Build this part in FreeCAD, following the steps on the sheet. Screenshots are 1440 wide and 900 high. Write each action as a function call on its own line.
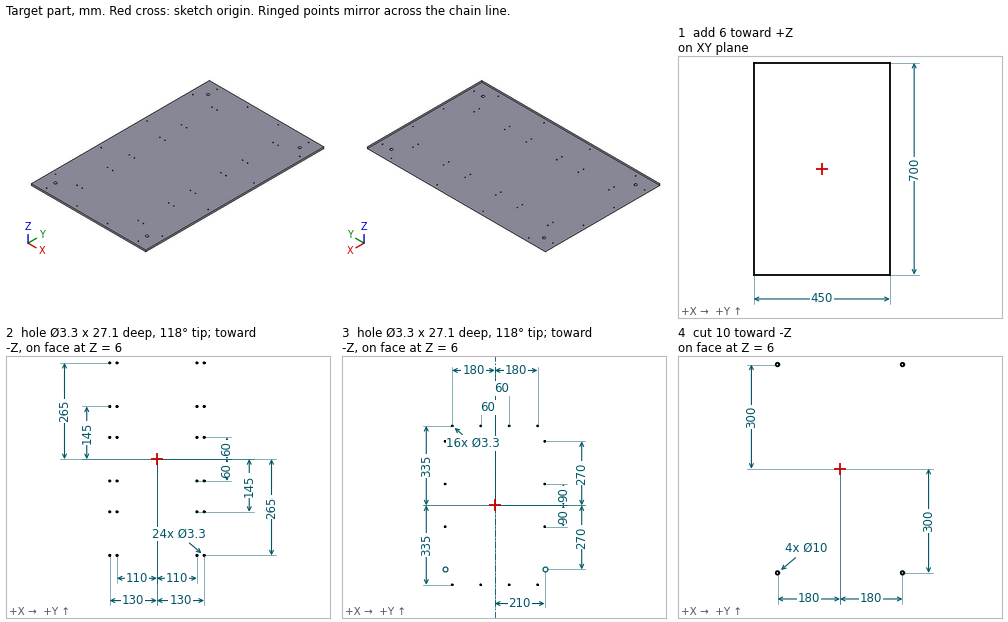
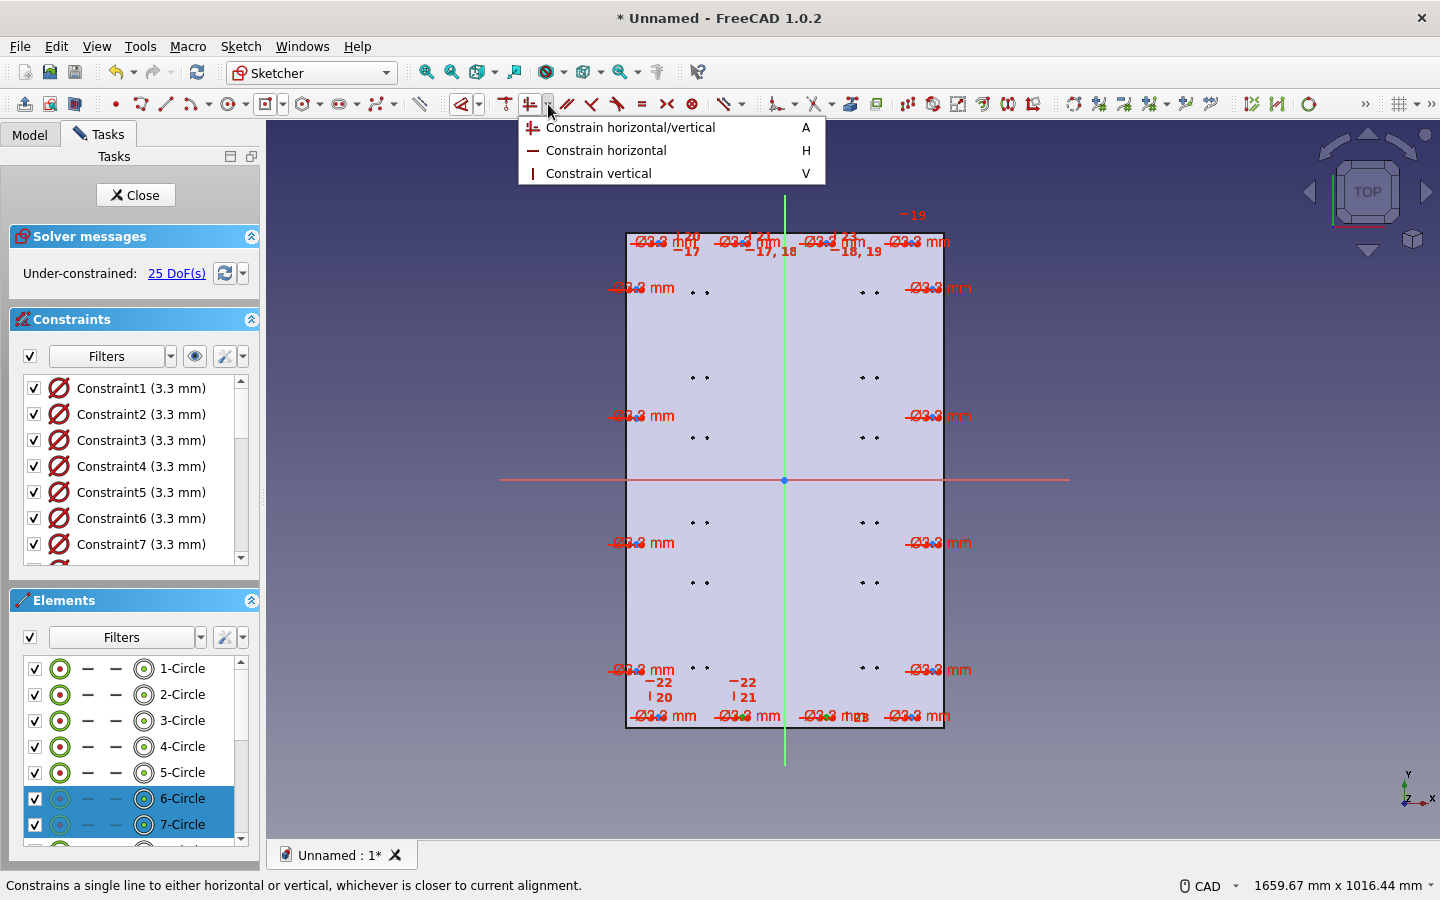
click(672, 150)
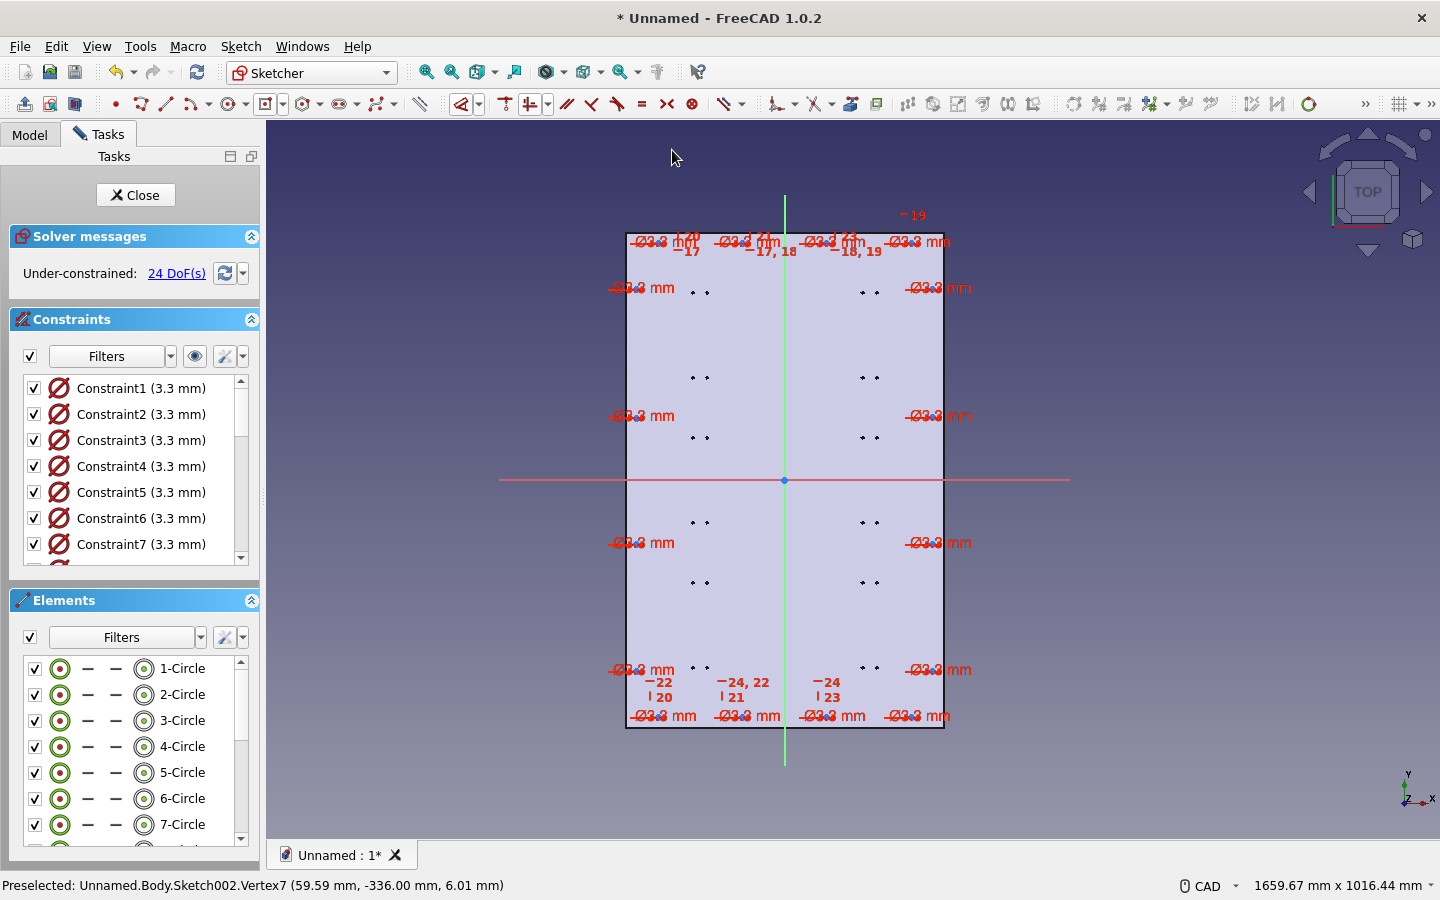
click(912, 244)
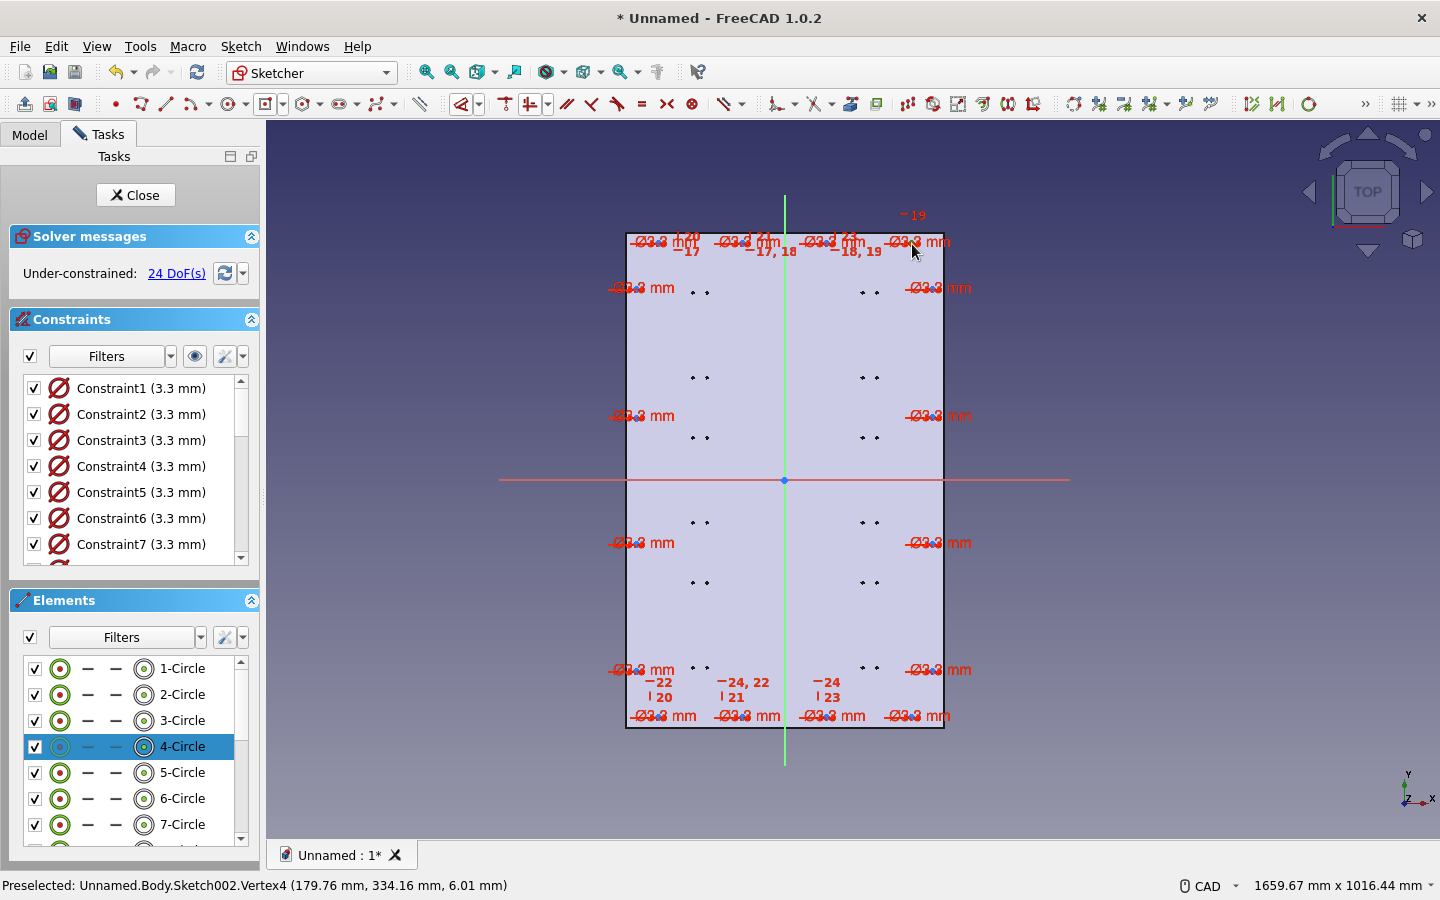
click(912, 718)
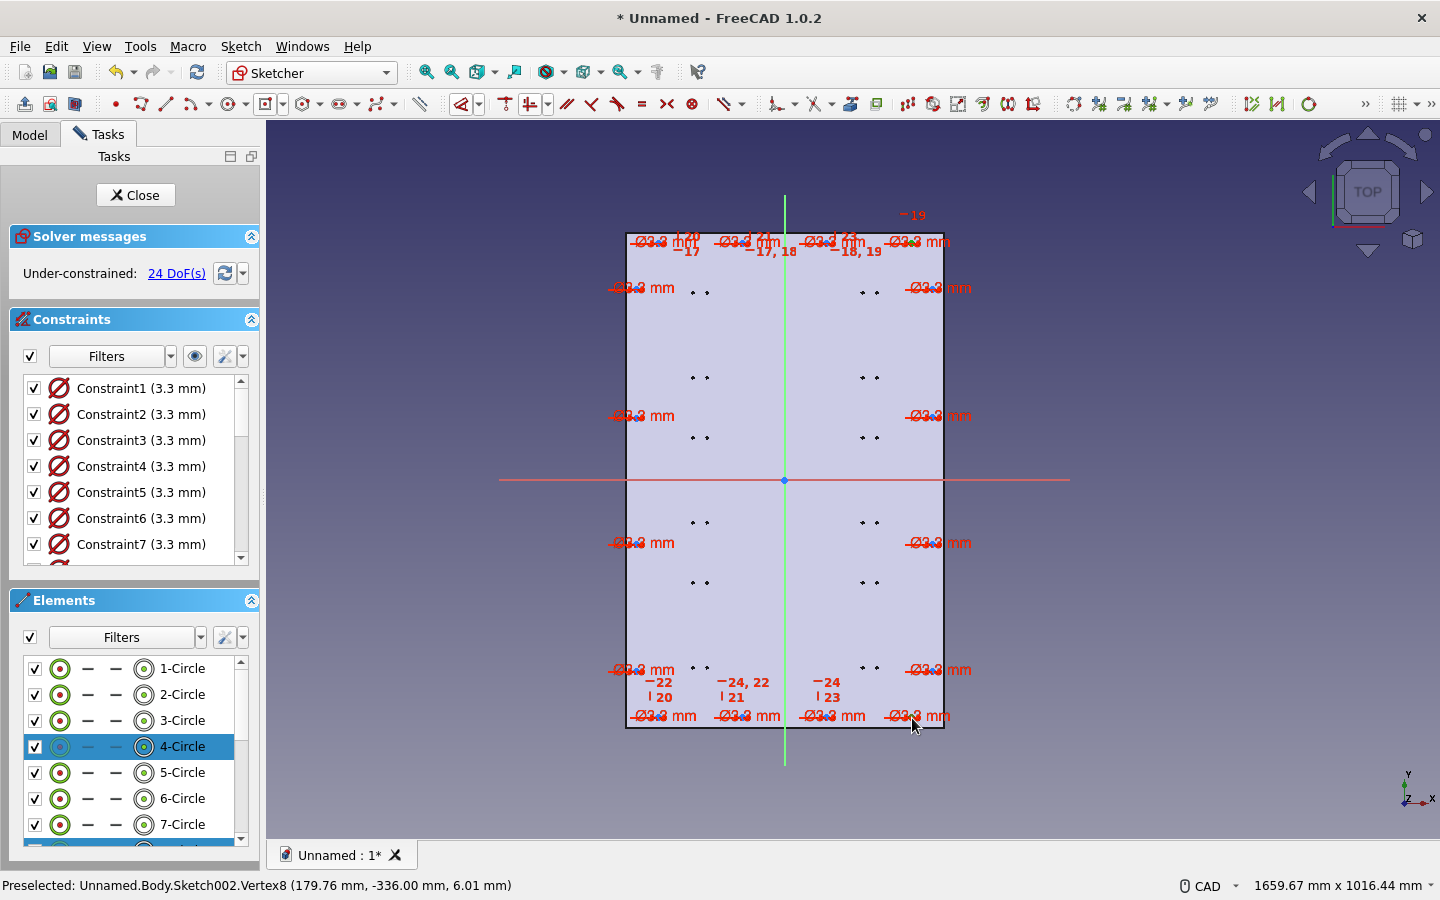
click(548, 104)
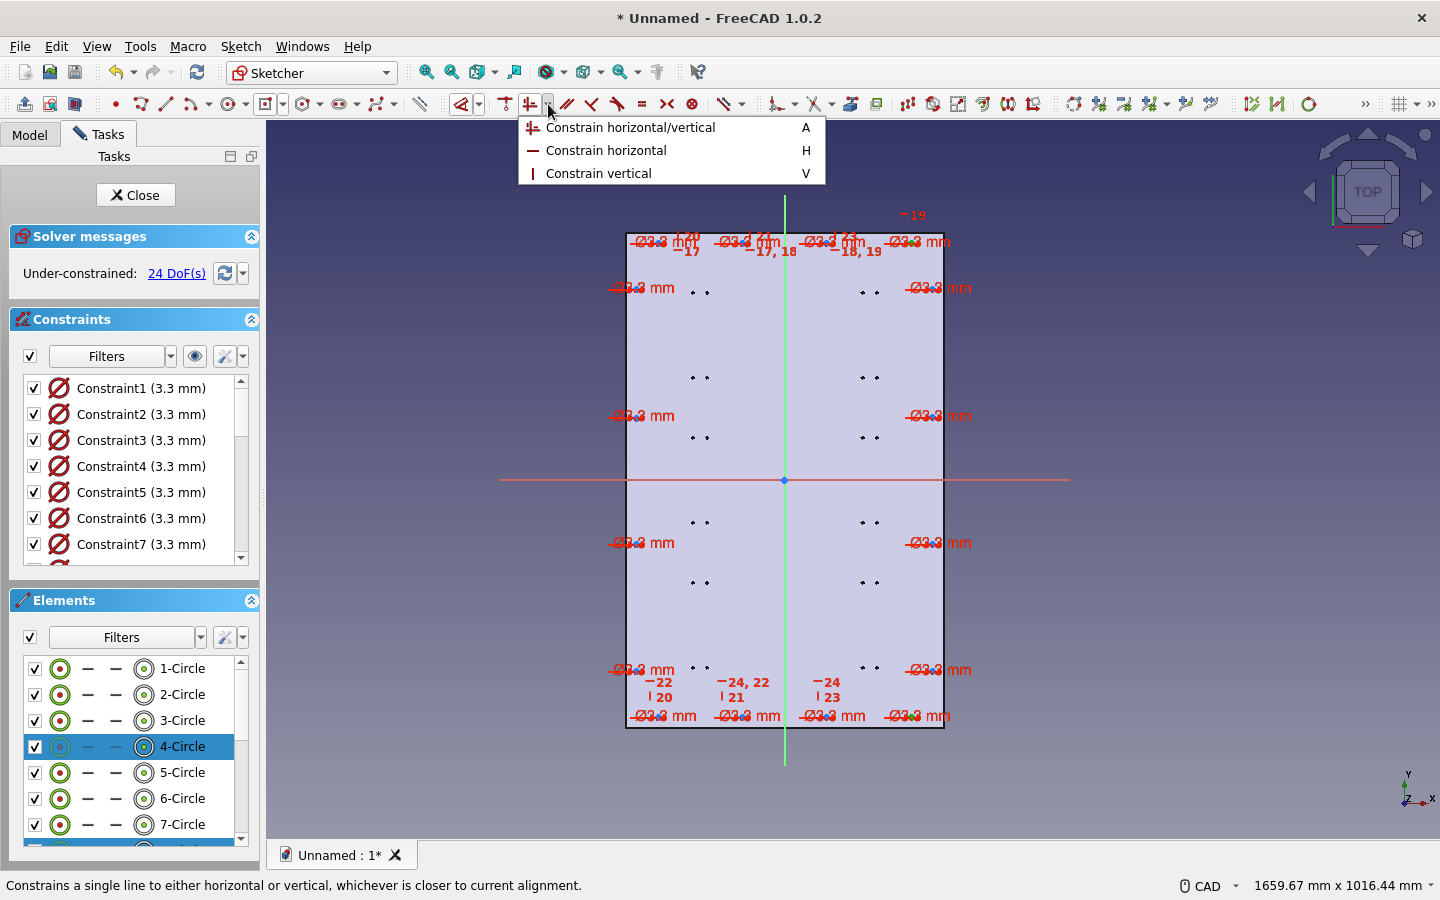
click(672, 174)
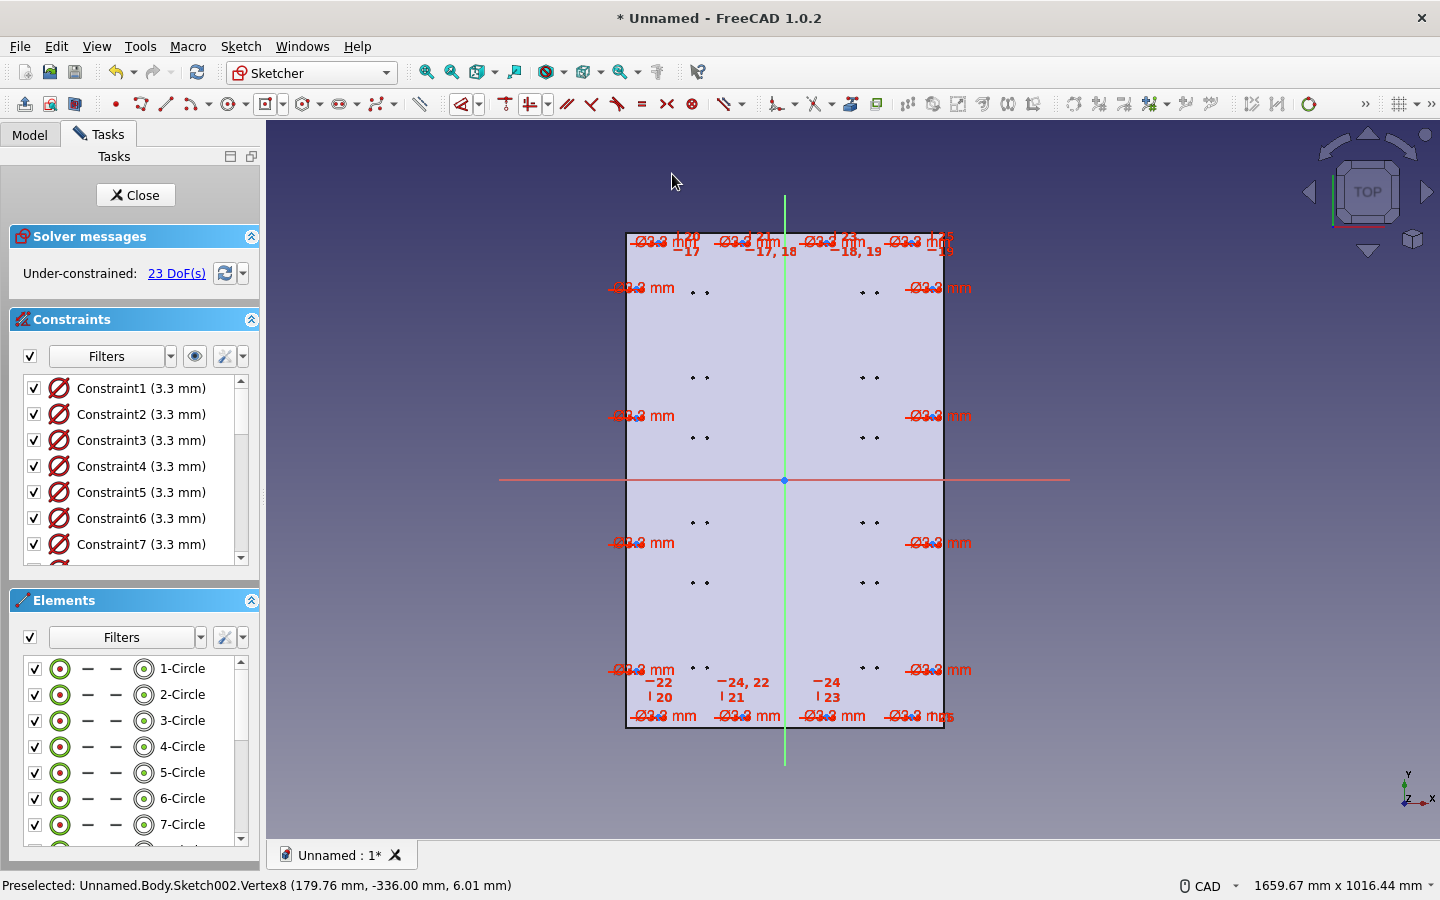
click(827, 718)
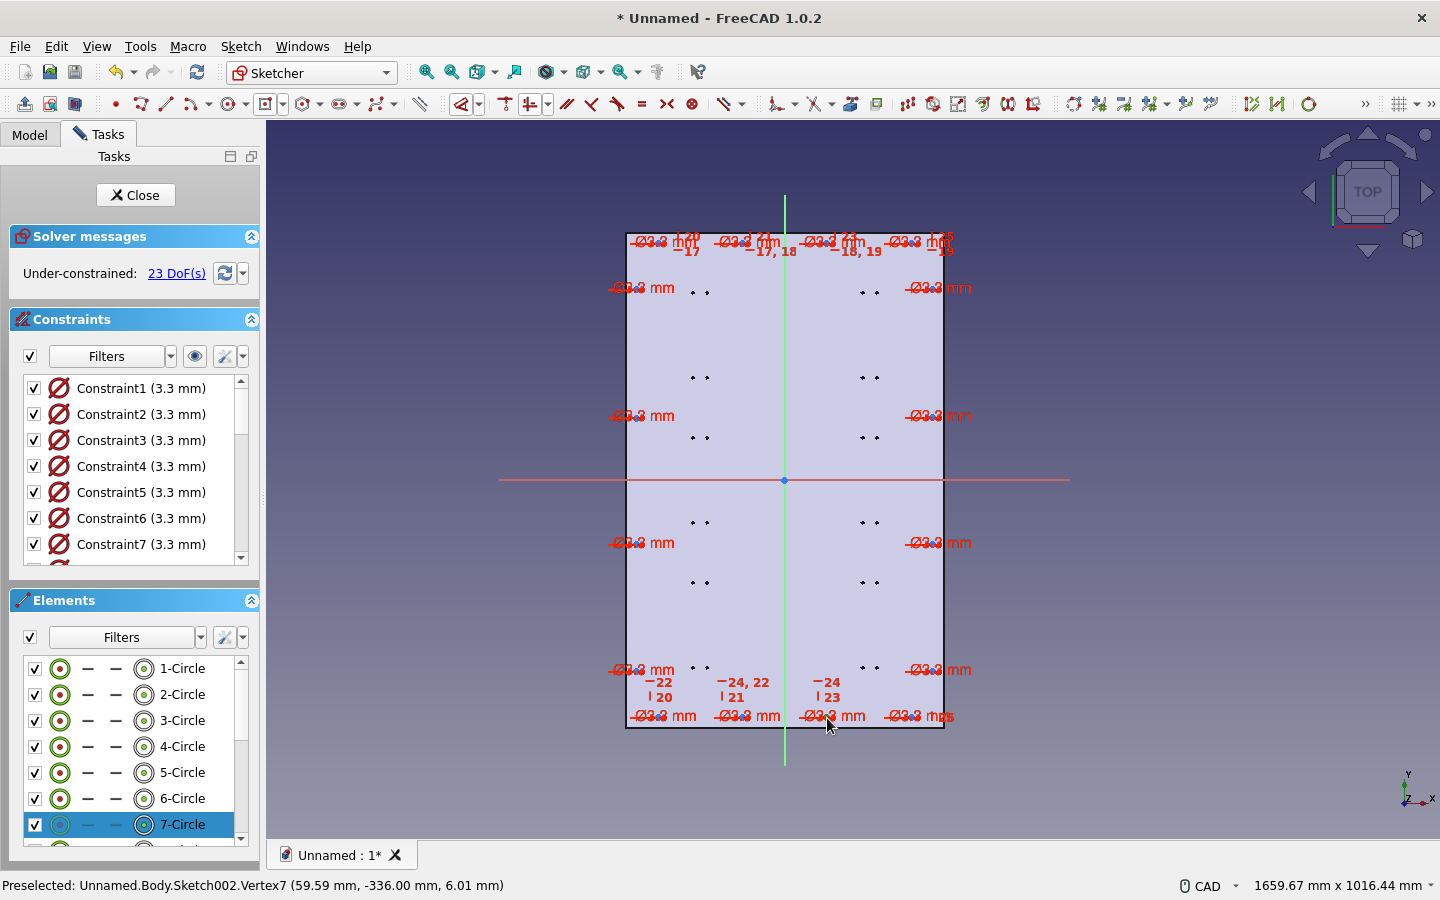
click(912, 718)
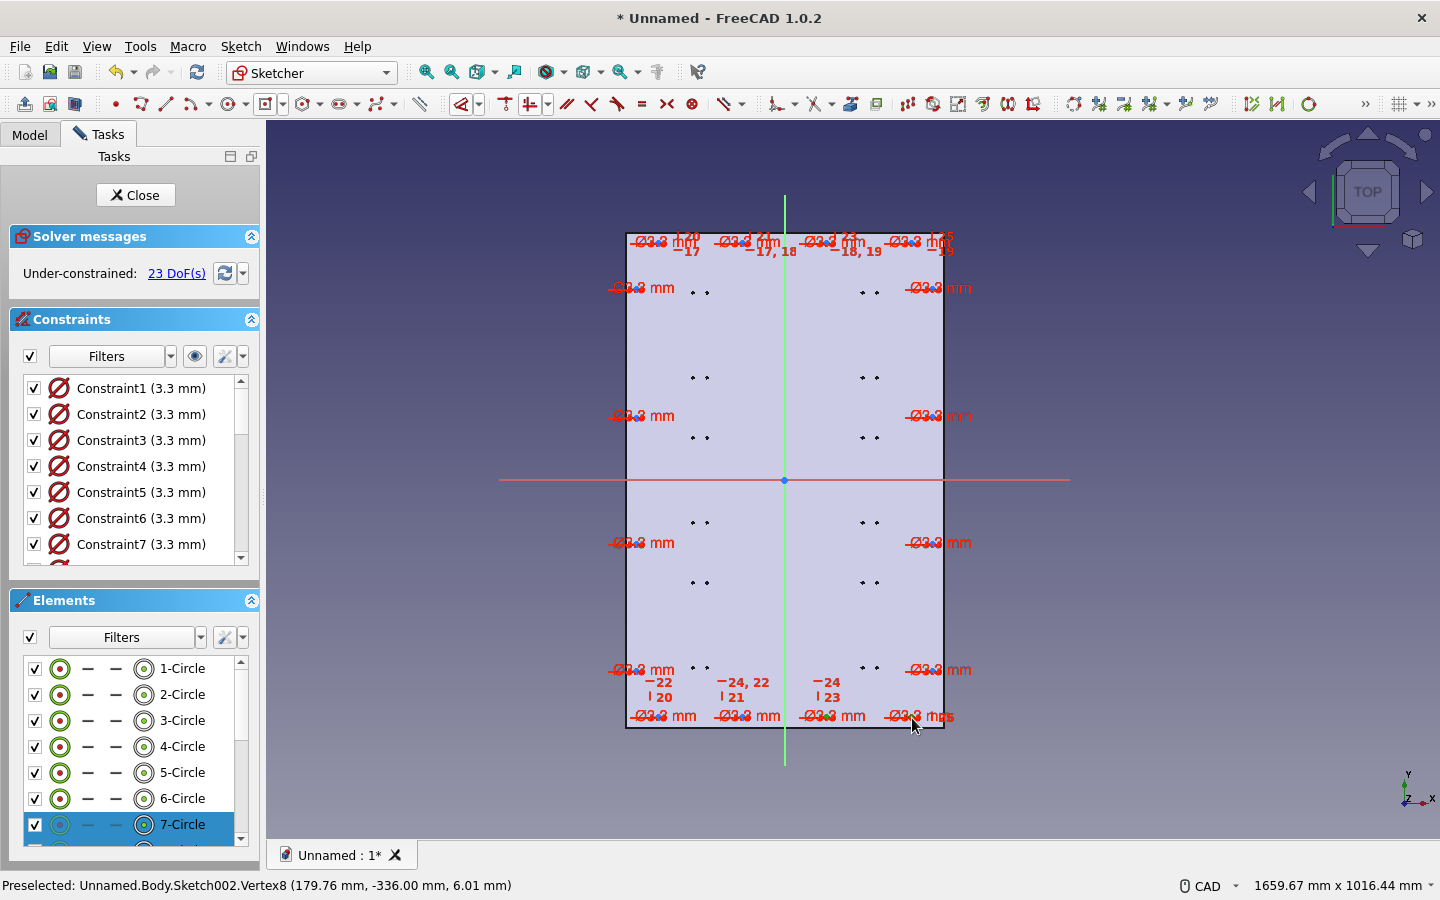
key(h)